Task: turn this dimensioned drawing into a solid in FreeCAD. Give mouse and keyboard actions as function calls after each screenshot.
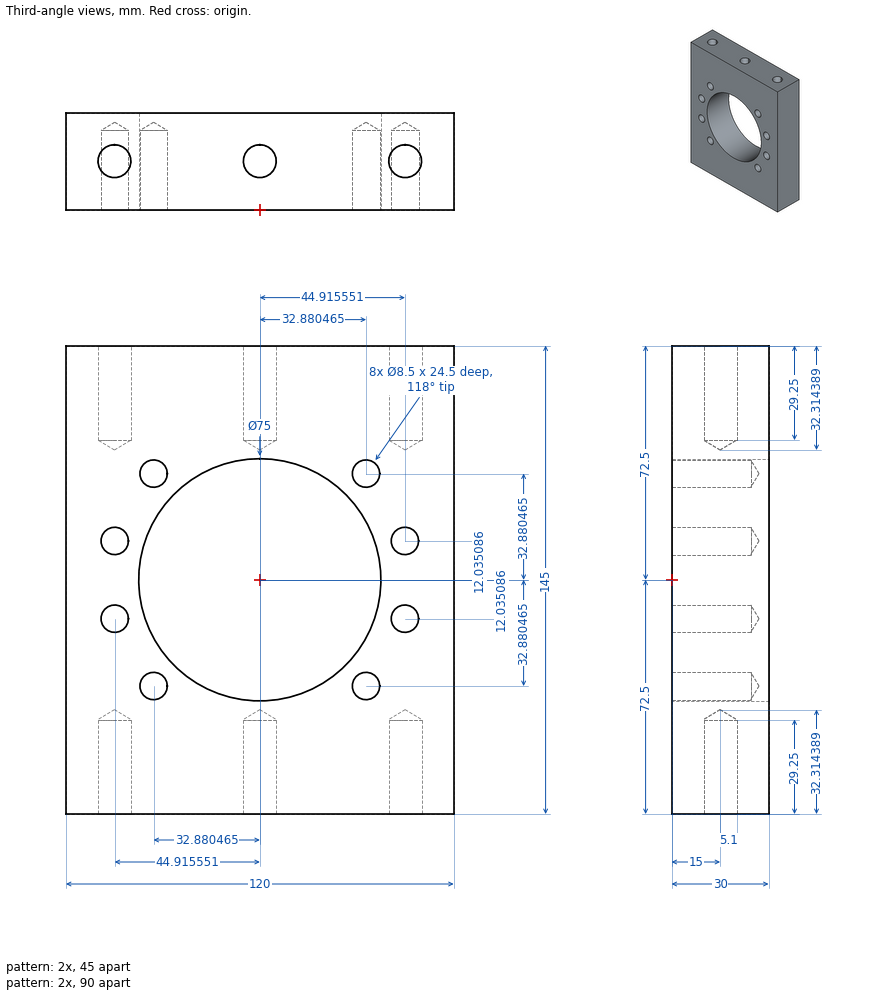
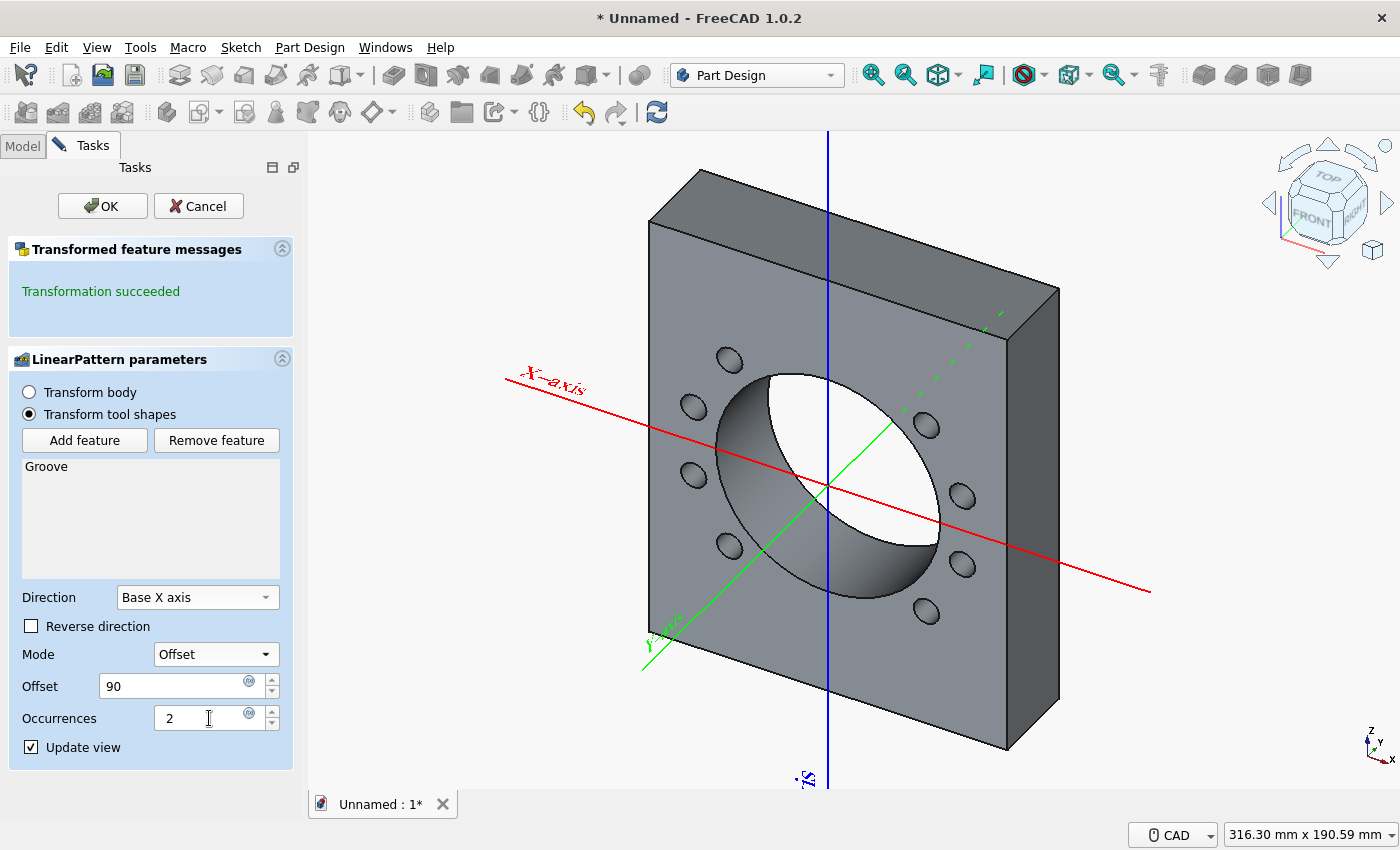
click(103, 206)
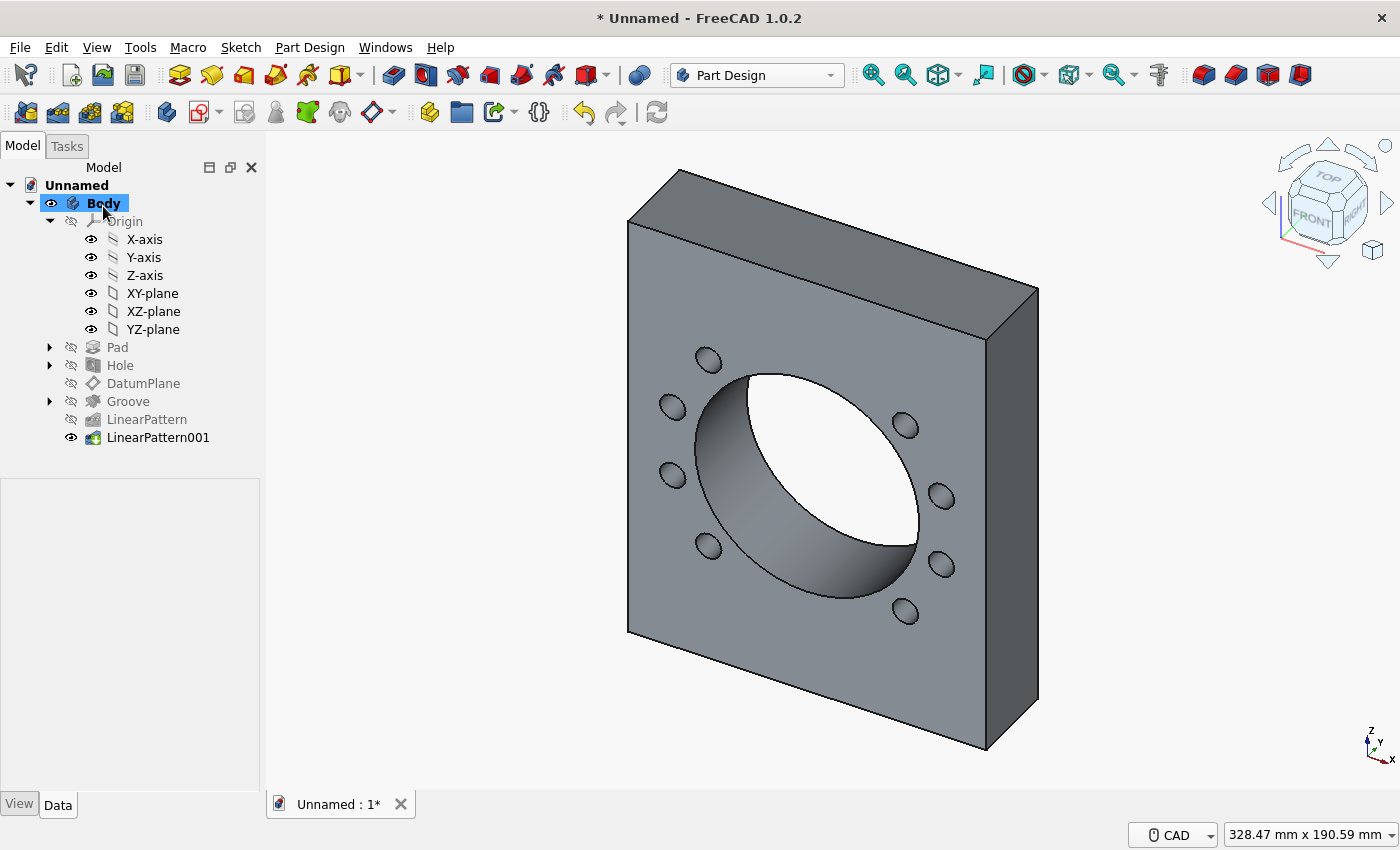
click(116, 401)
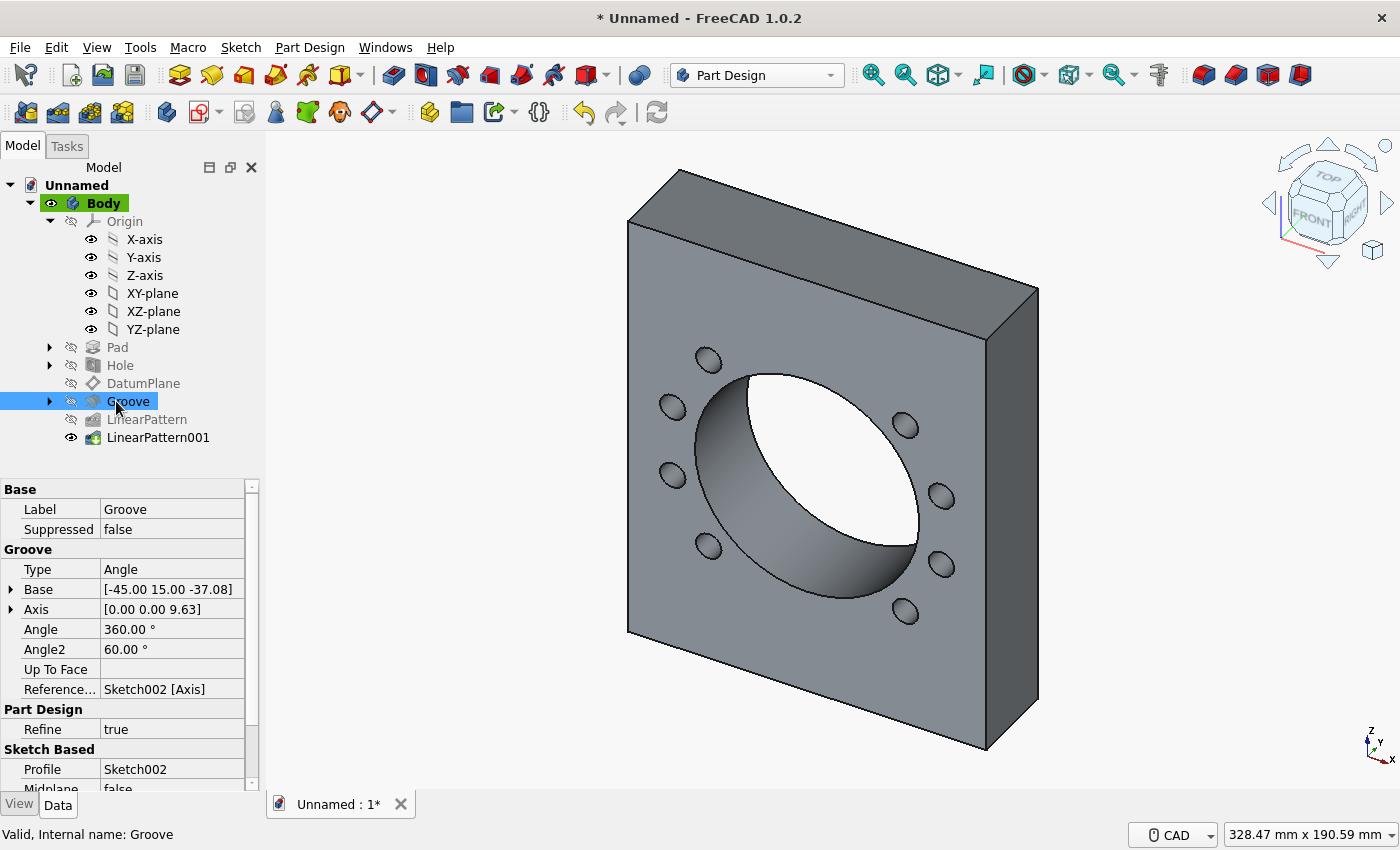
click(26, 112)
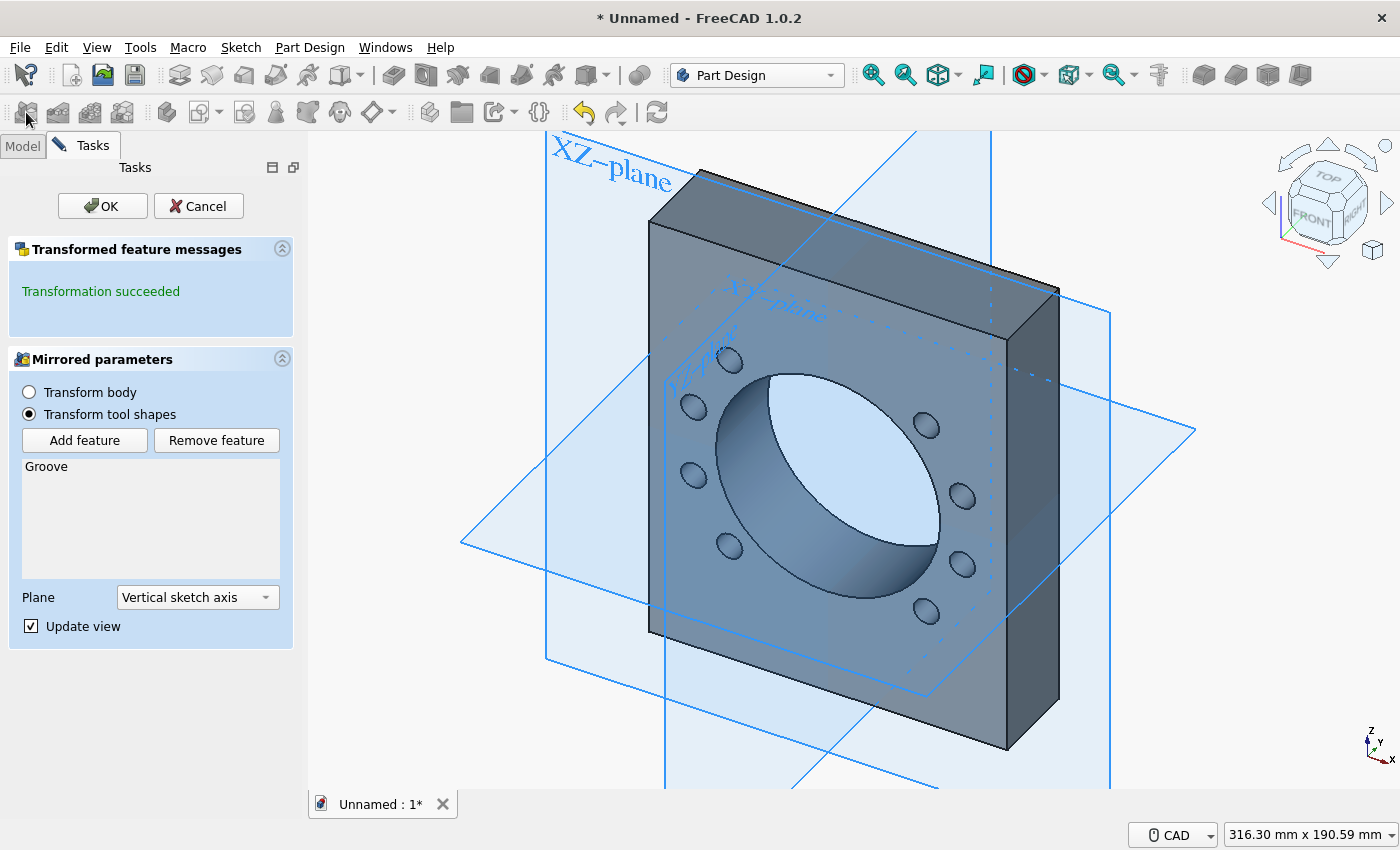
click(198, 598)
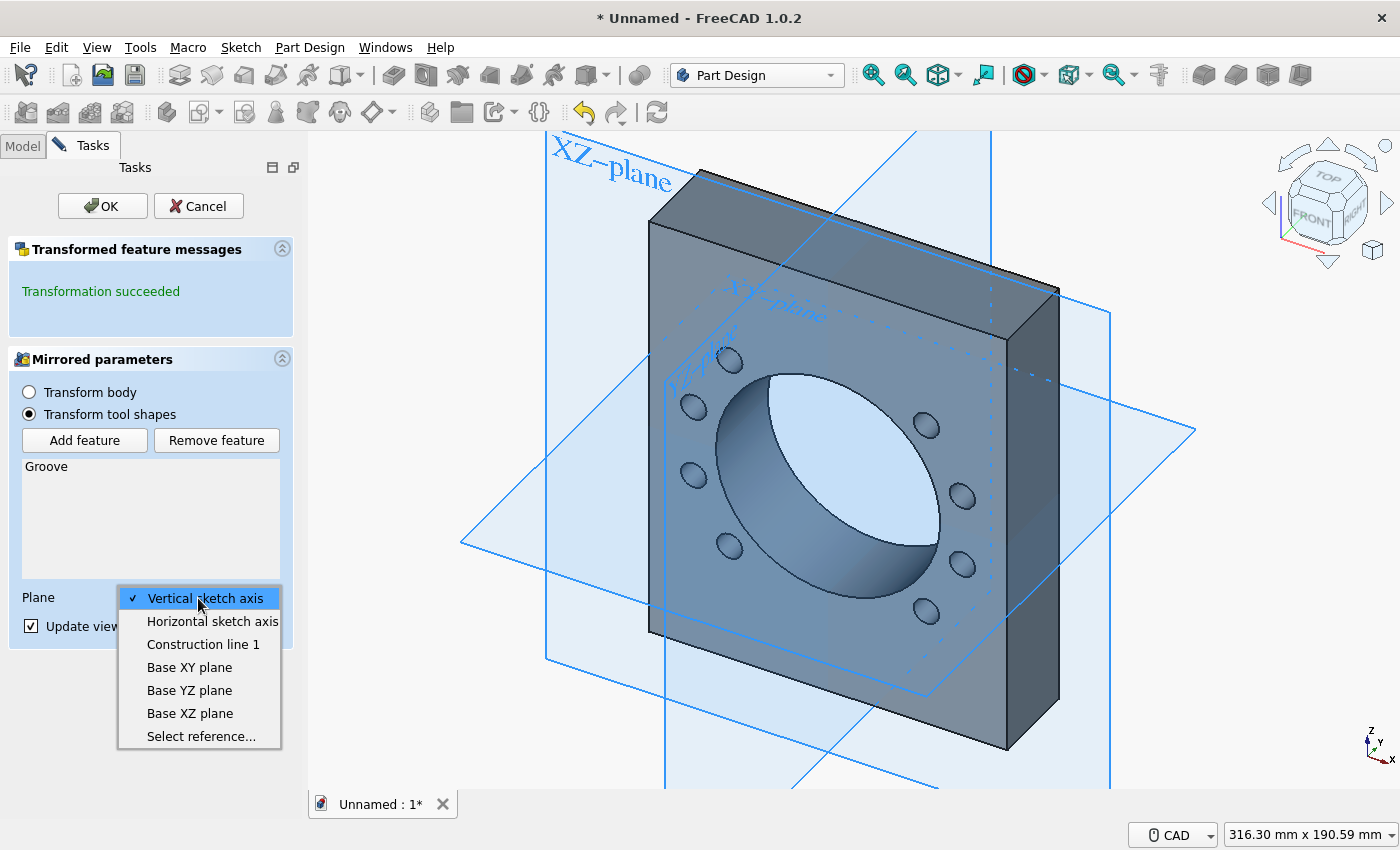
click(198, 668)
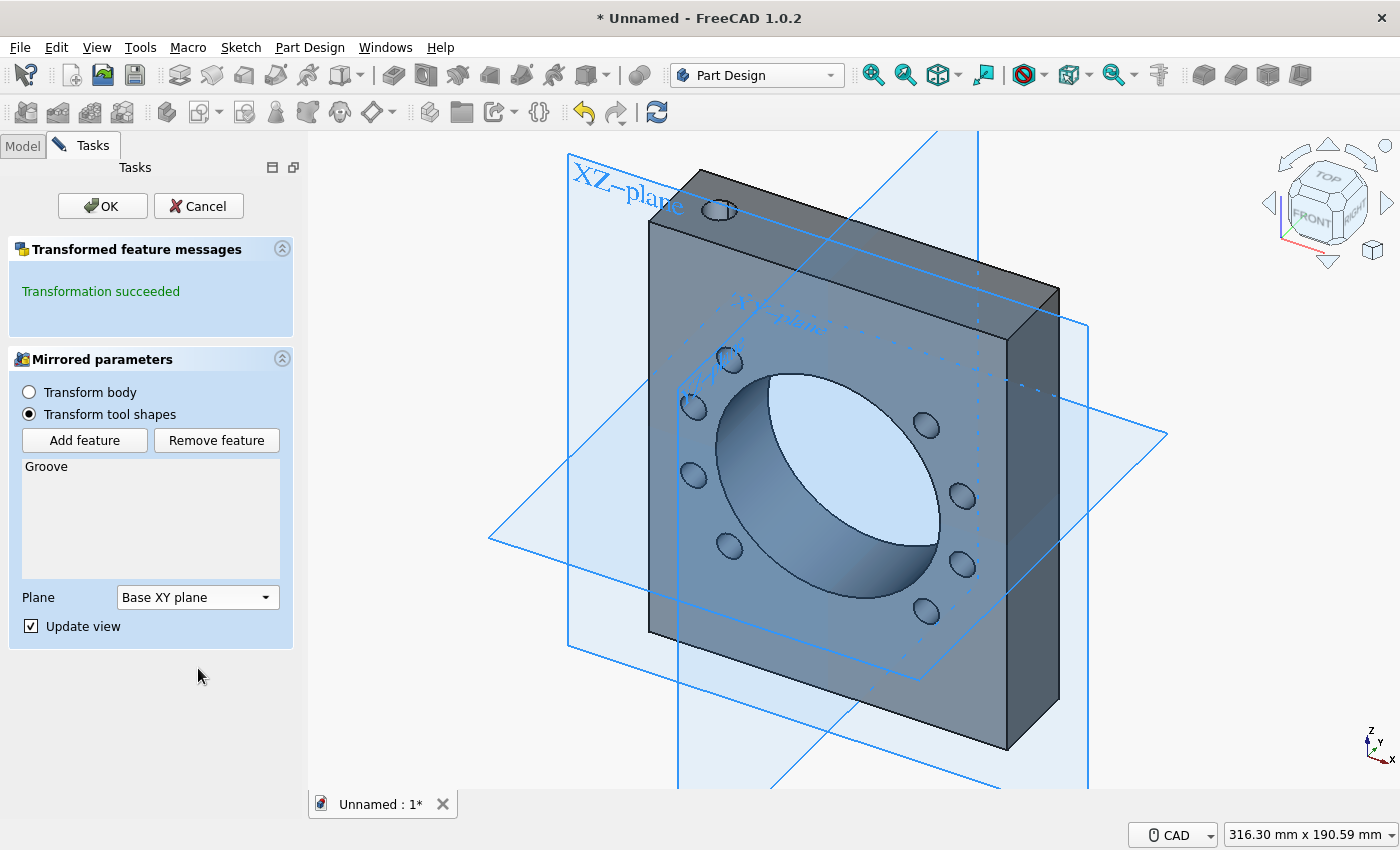
click(103, 206)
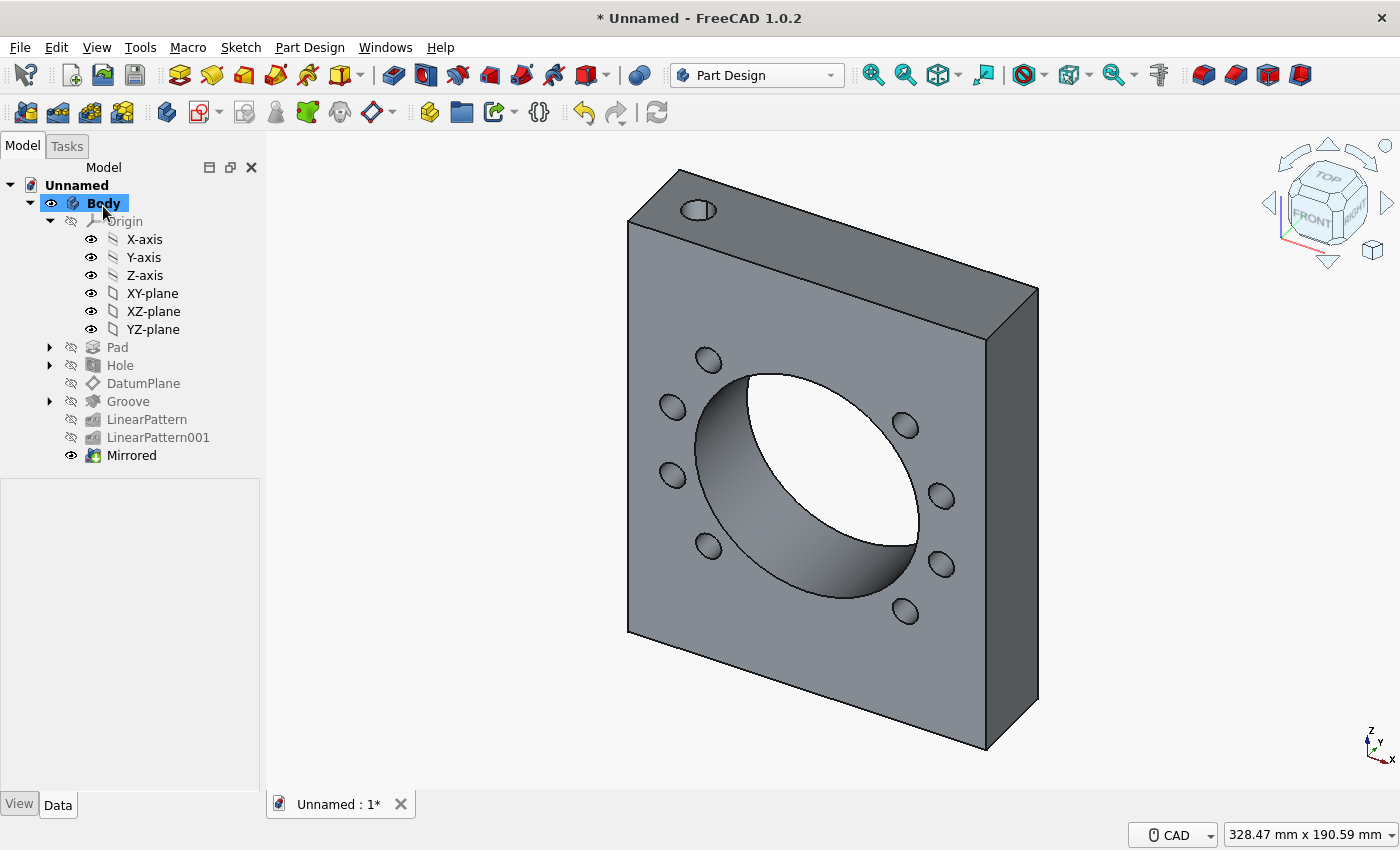
click(200, 112)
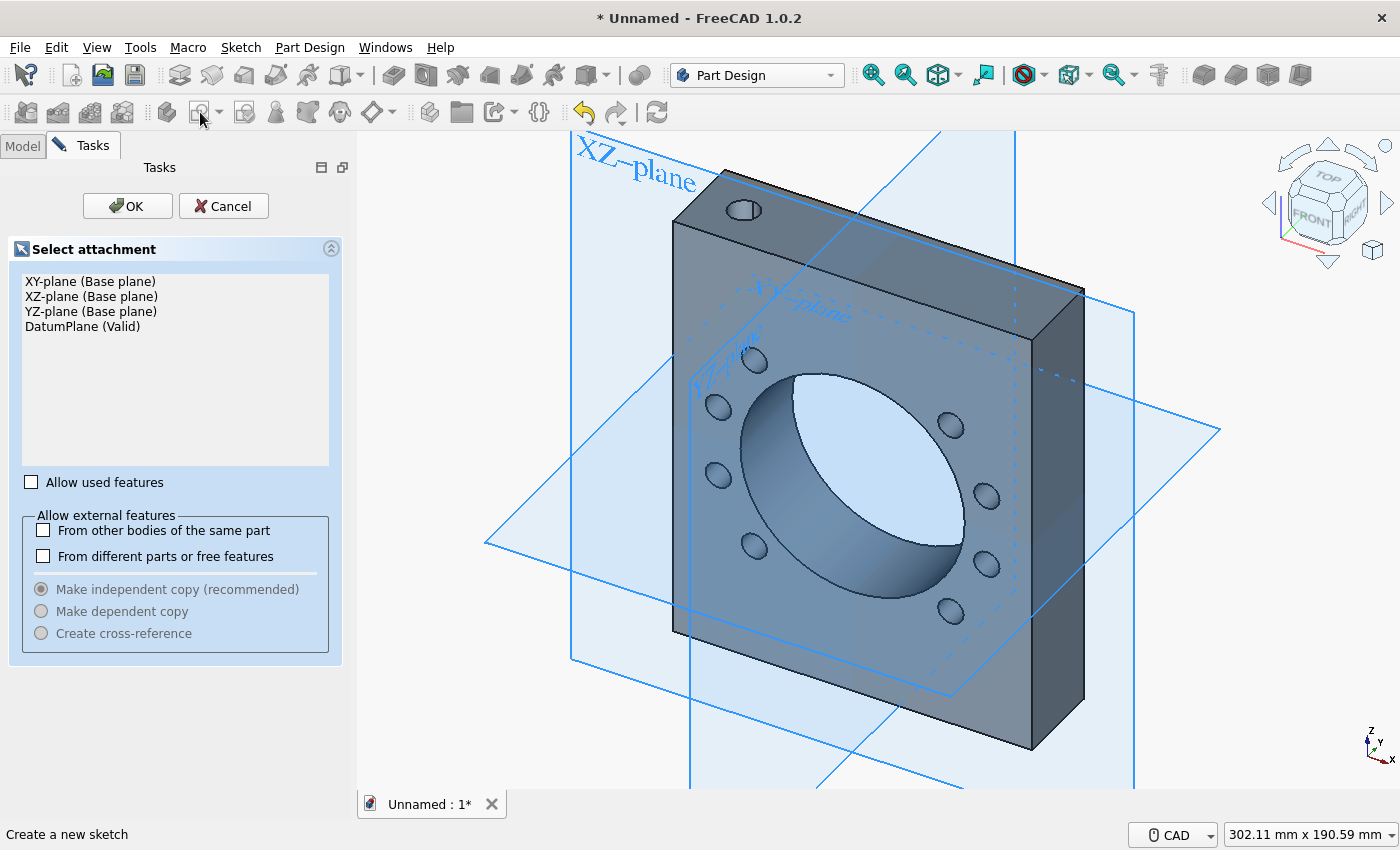
click(82, 312)